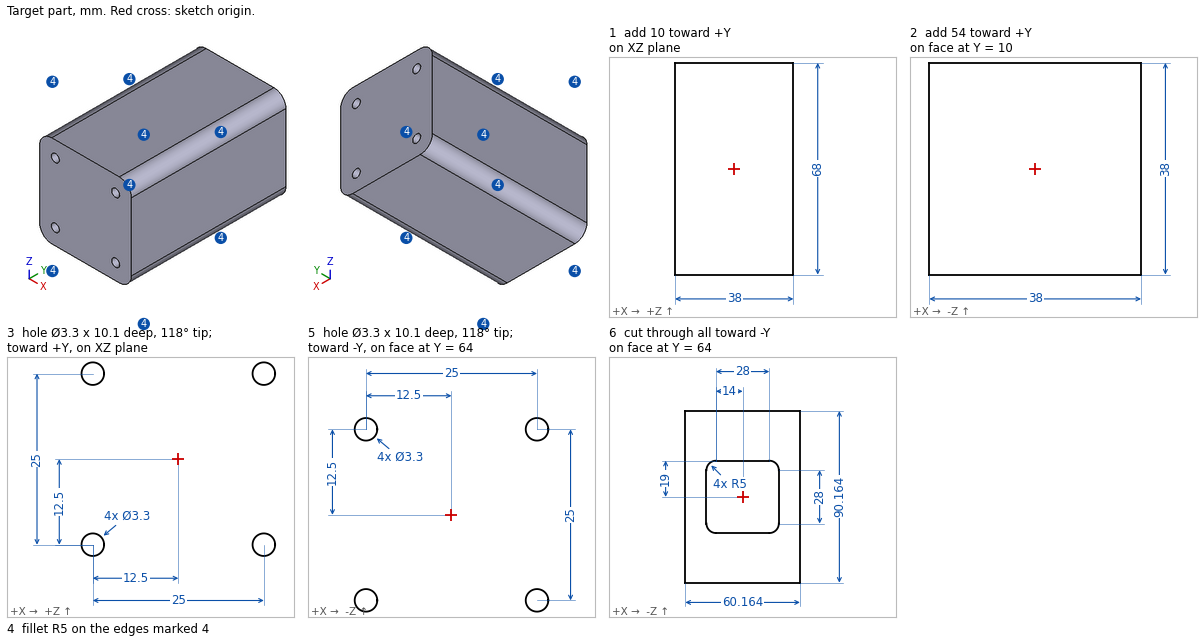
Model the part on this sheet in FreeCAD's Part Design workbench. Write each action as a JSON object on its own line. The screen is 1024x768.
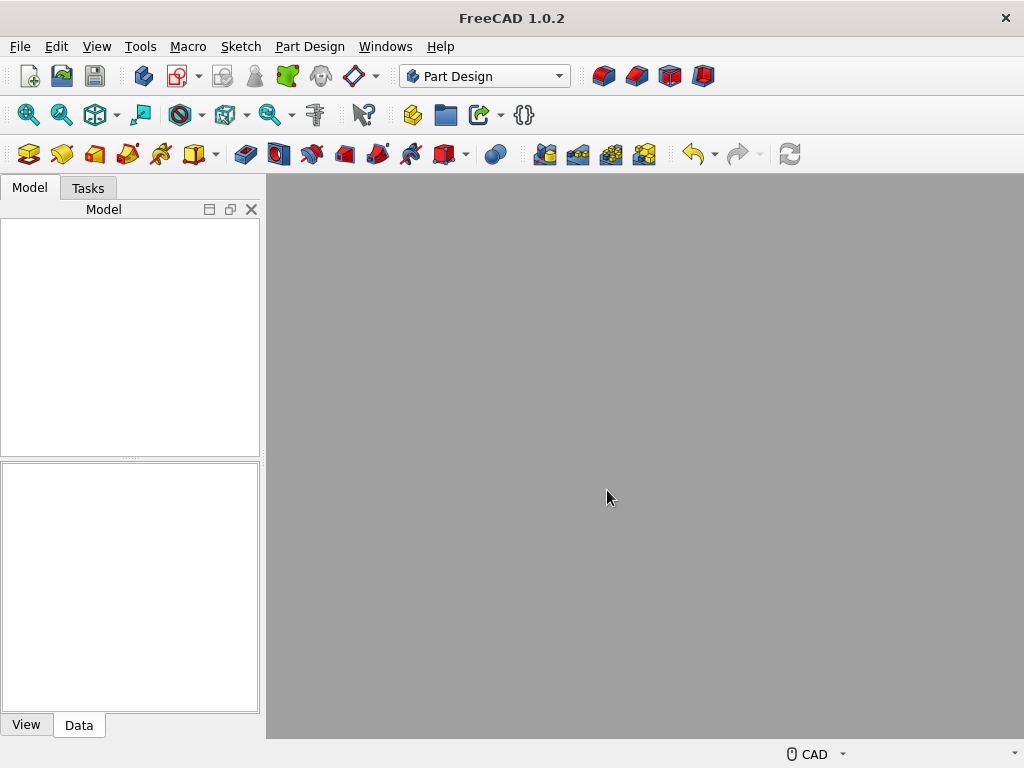
{"action": "left_click", "coordinate": [29, 76]}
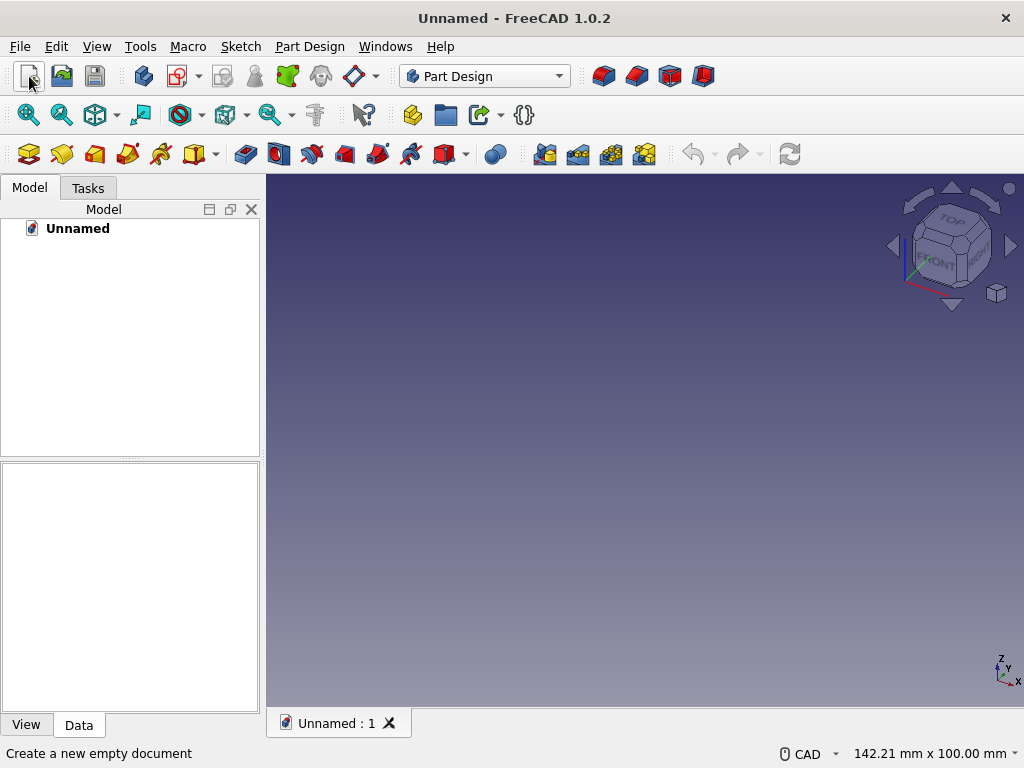
{"action": "left_click", "coordinate": [176, 76]}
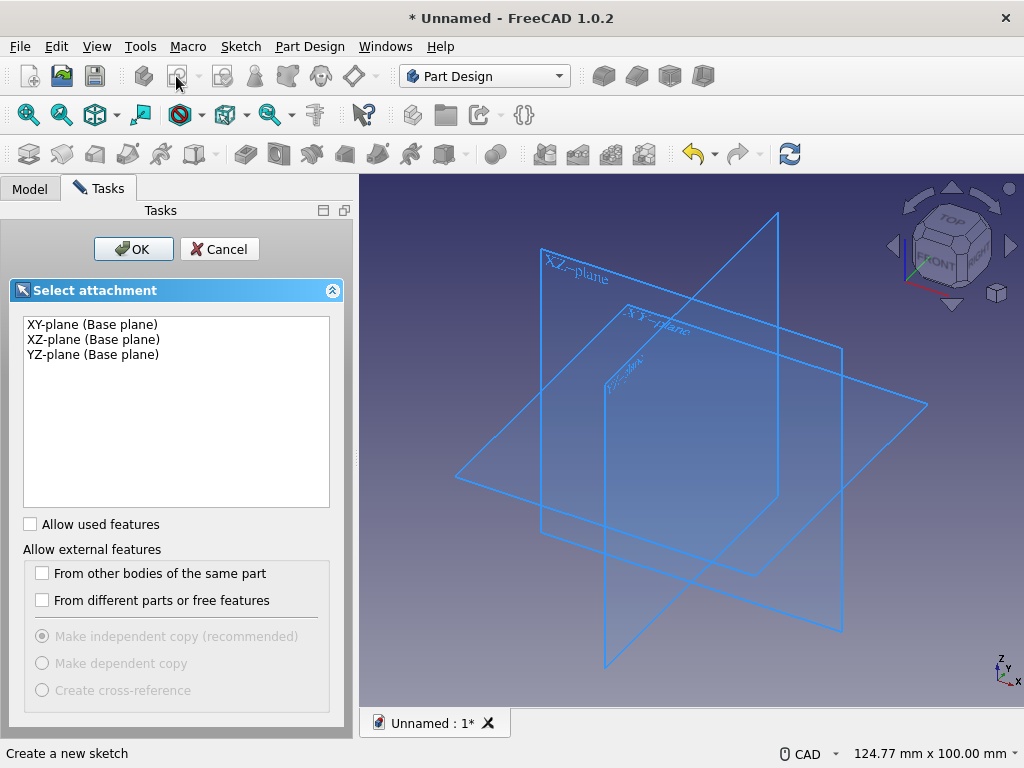
{"action": "left_click", "coordinate": [84, 340]}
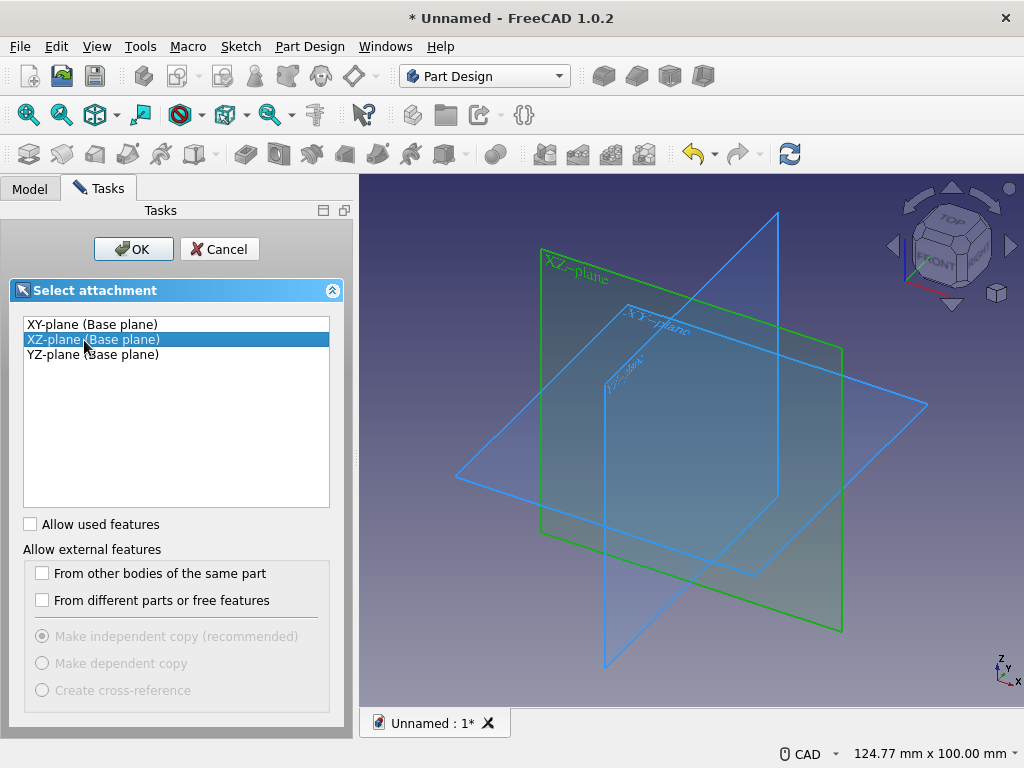
{"action": "left_click", "coordinate": [134, 249]}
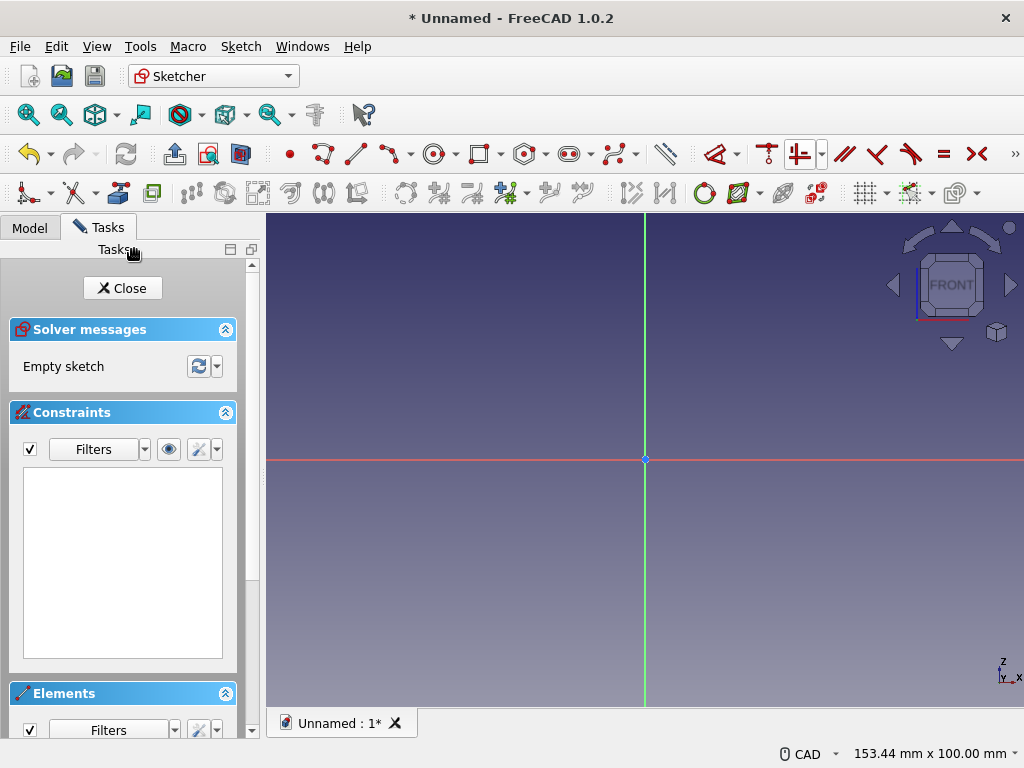
{"action": "left_click", "coordinate": [500, 154]}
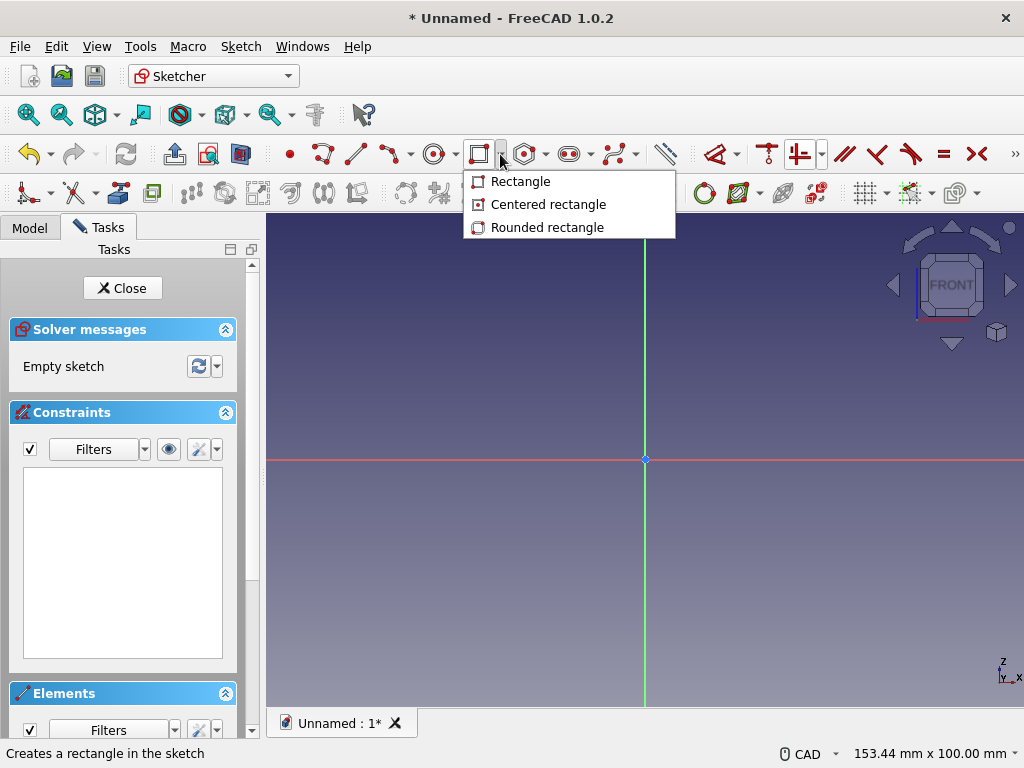
{"action": "left_click", "coordinate": [570, 204]}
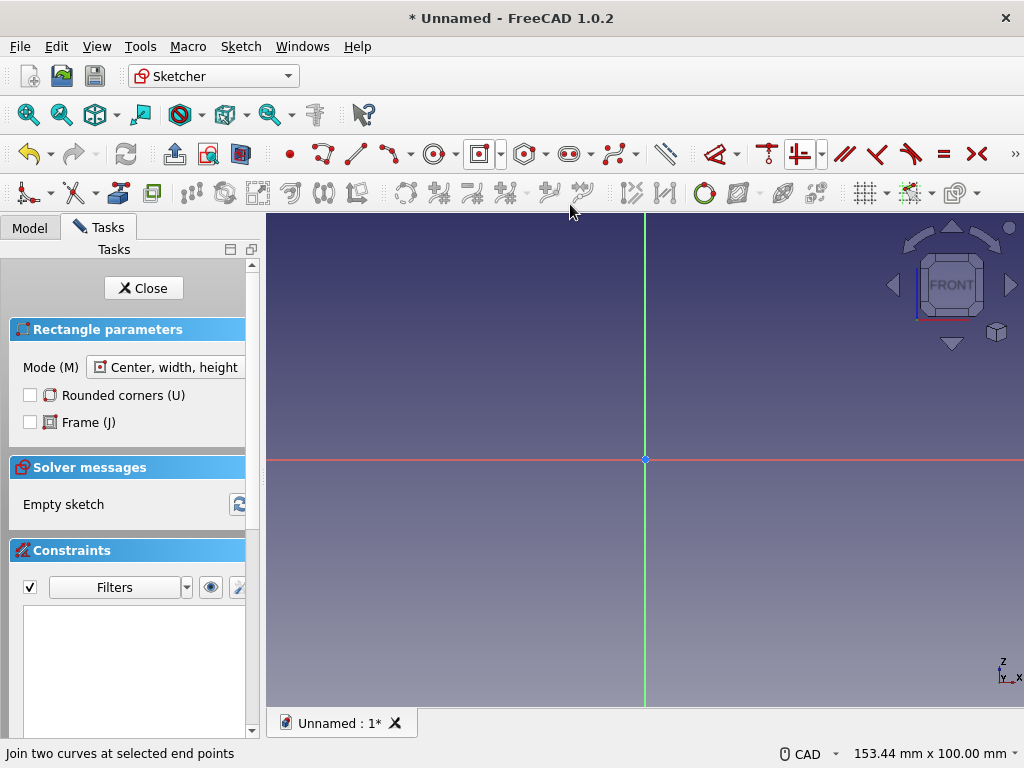
{"action": "left_click", "coordinate": [645, 460]}
{"action": "left_click", "coordinate": [739, 292]}
{"action": "key", "text": "Escape"}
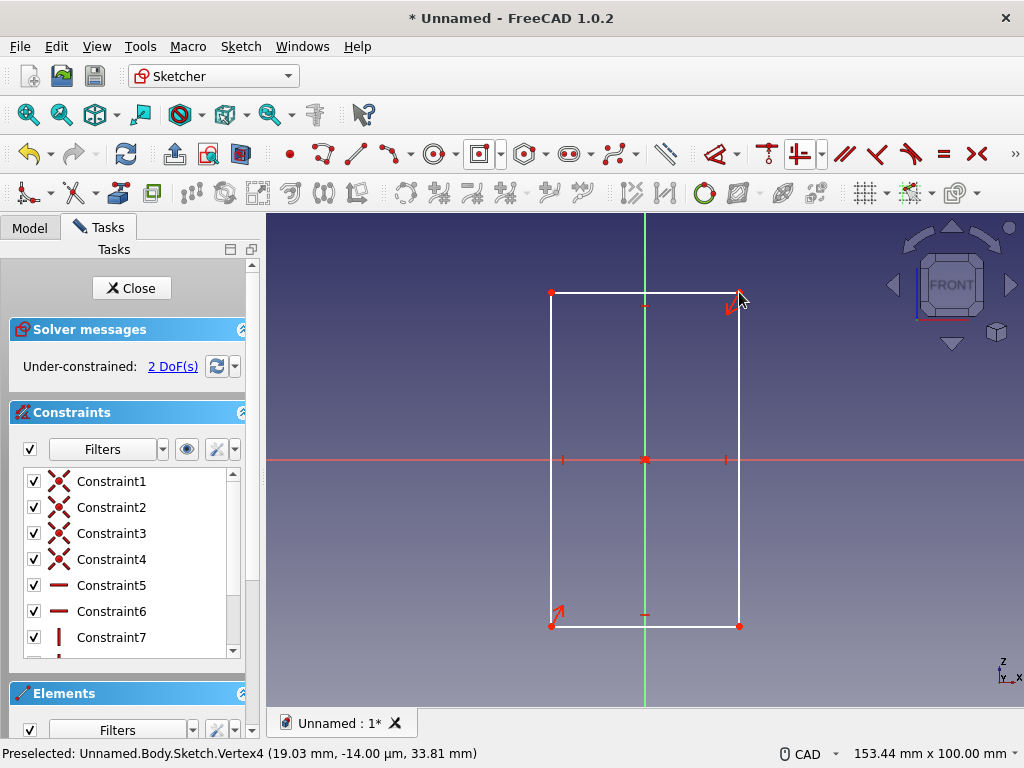
{"action": "left_click", "coordinate": [714, 154]}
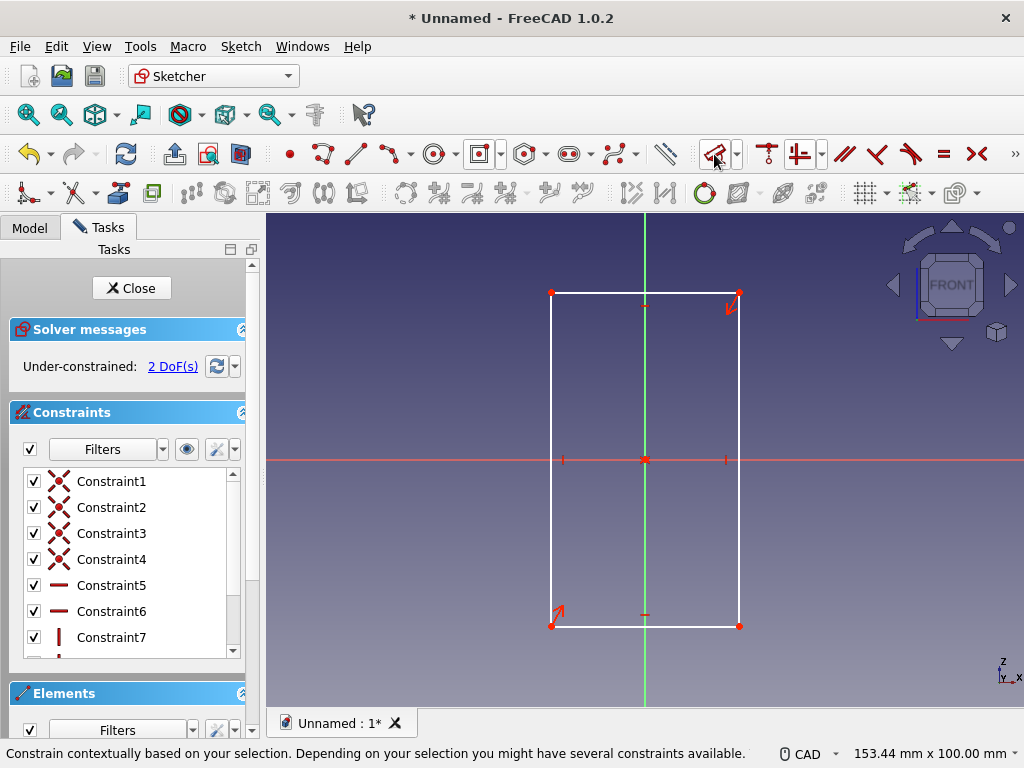
{"action": "left_click", "coordinate": [607, 627]}
{"action": "left_click", "coordinate": [602, 661]}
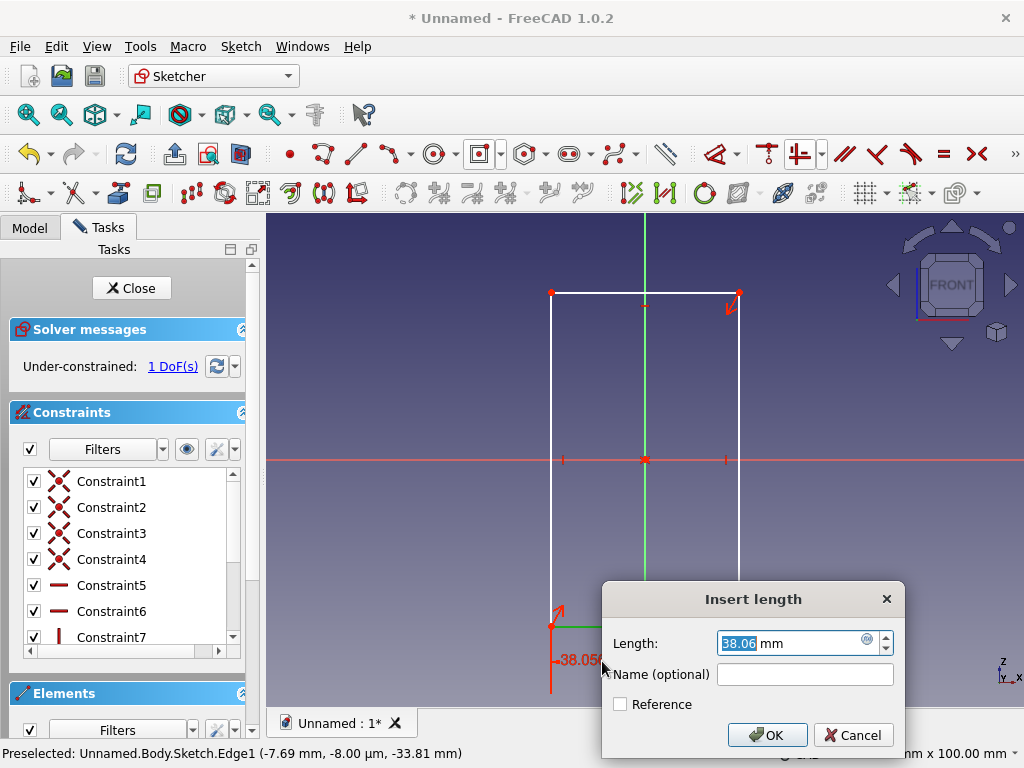
{"action": "type", "text": "38"}
{"action": "key", "text": "Return"}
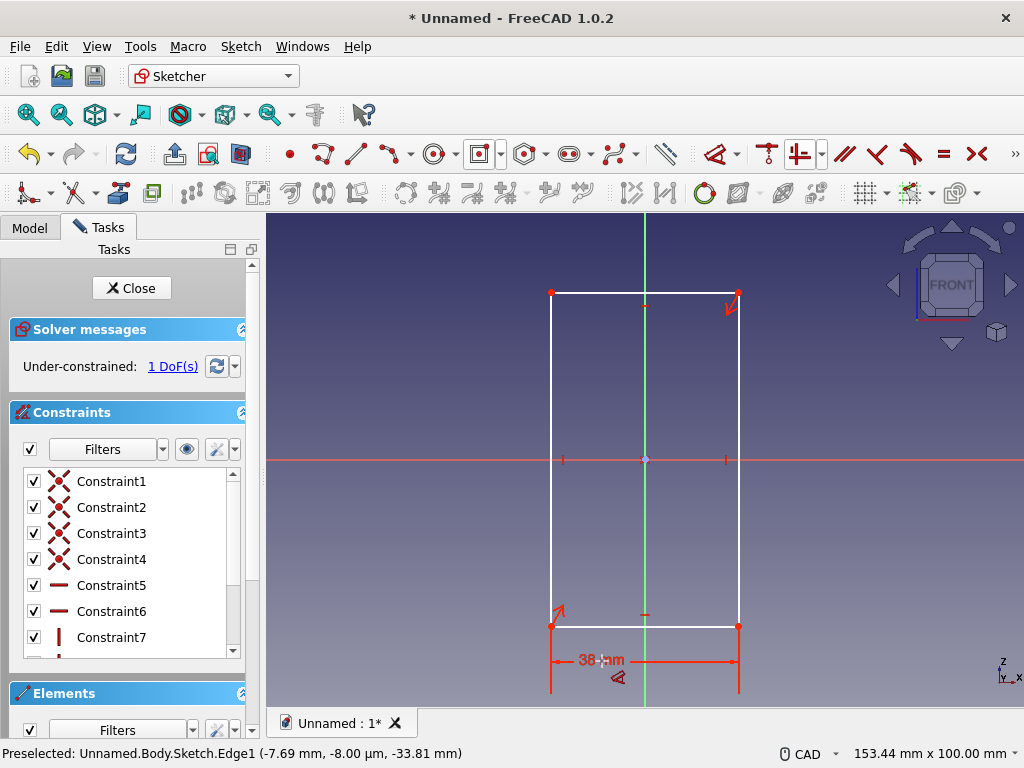
{"action": "left_click", "coordinate": [739, 527]}
{"action": "left_click", "coordinate": [773, 383]}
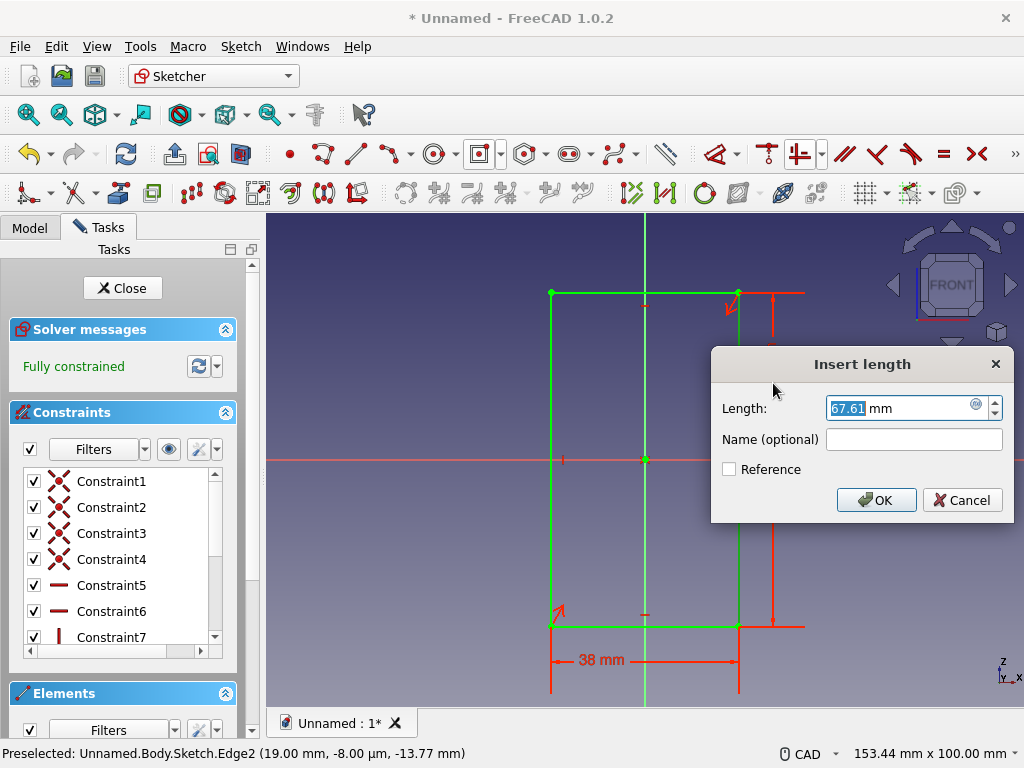
{"action": "type", "text": "68"}
{"action": "key", "text": "Return"}
{"action": "key", "text": "Escape"}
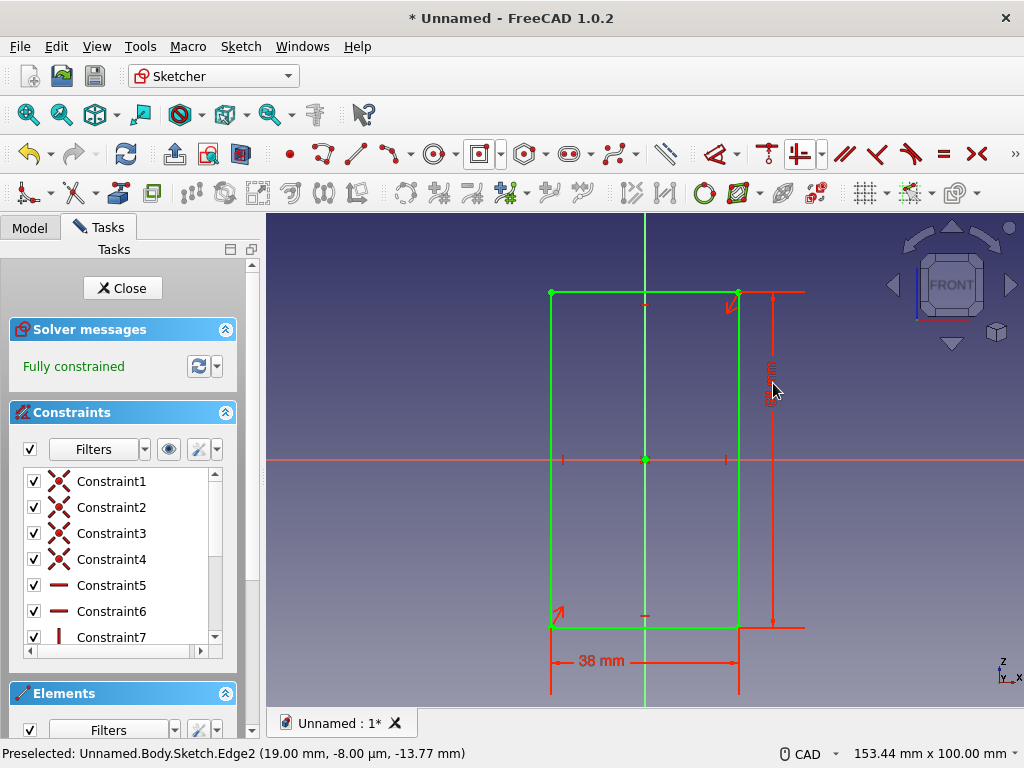
{"action": "left_click", "coordinate": [123, 288]}